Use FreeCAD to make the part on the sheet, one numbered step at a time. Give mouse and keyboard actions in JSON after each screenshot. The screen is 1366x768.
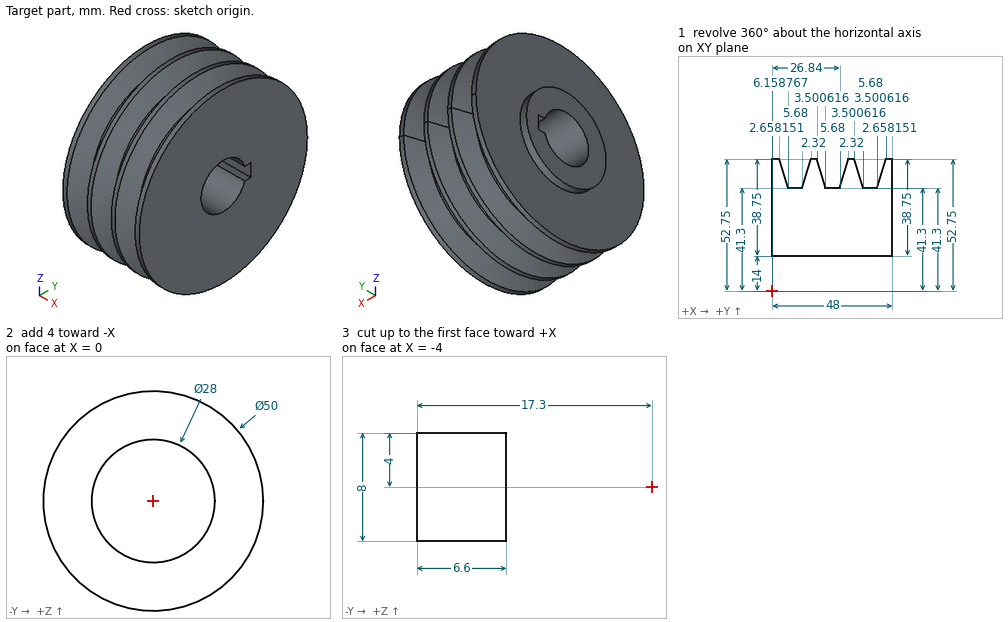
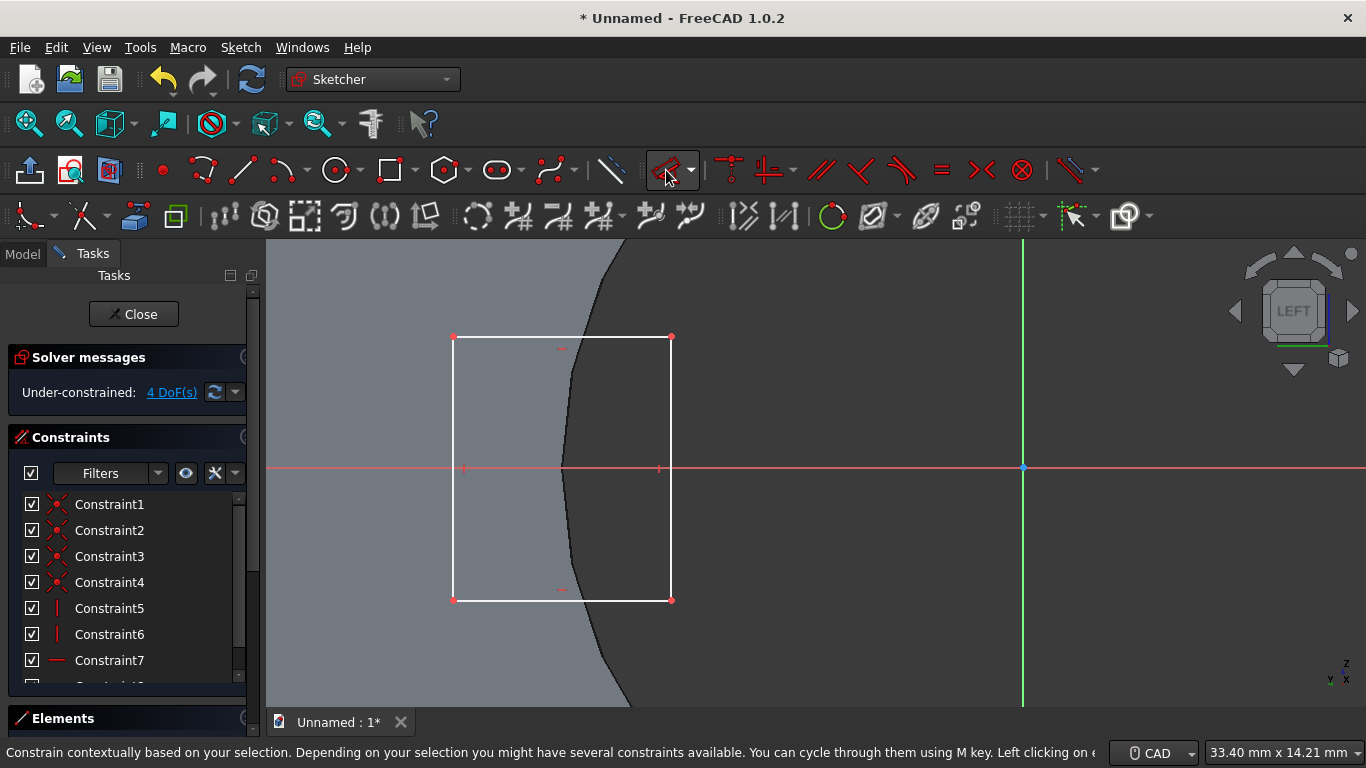
{"action": "left_click", "coordinate": [453, 416]}
{"action": "left_click", "coordinate": [419, 408]}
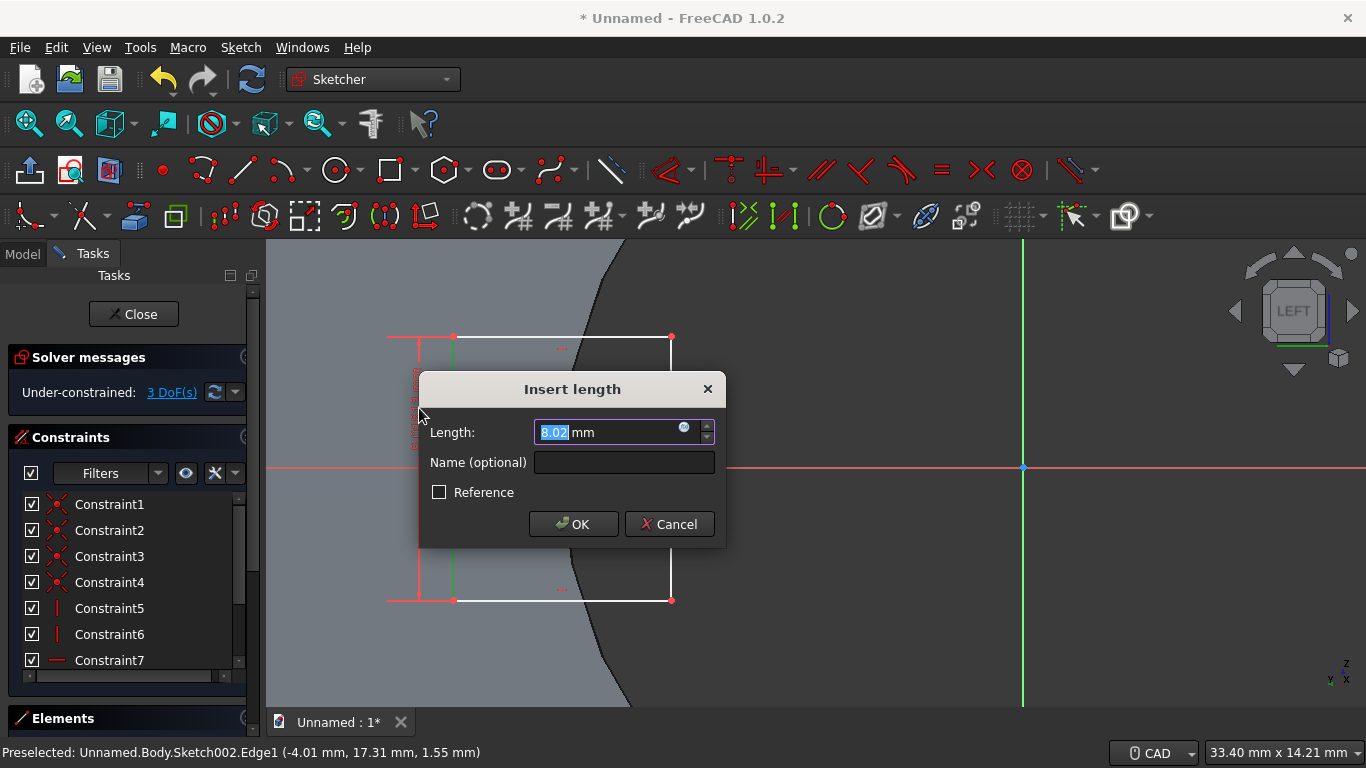
{"action": "type", "text": "8"}
{"action": "key", "text": "Return"}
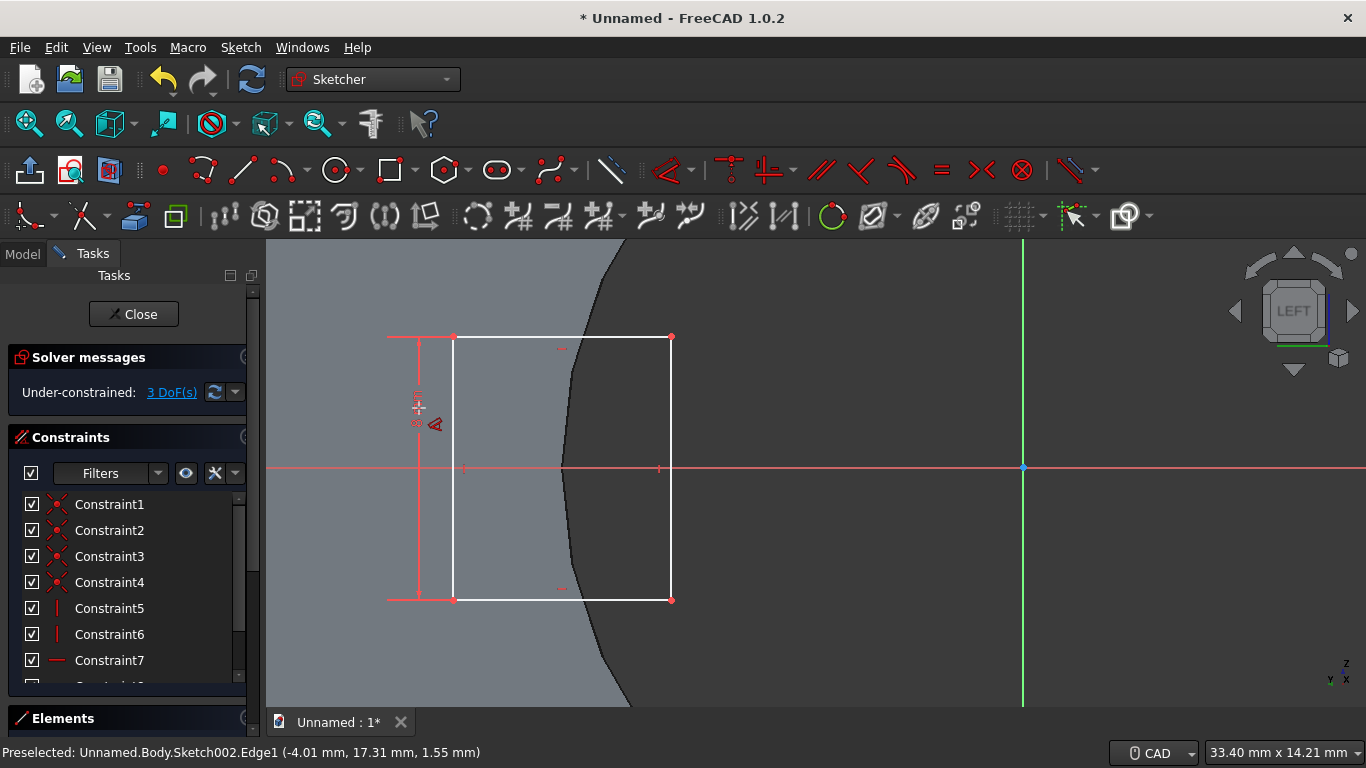
{"action": "left_click", "coordinate": [453, 337]}
{"action": "left_click", "coordinate": [419, 372]}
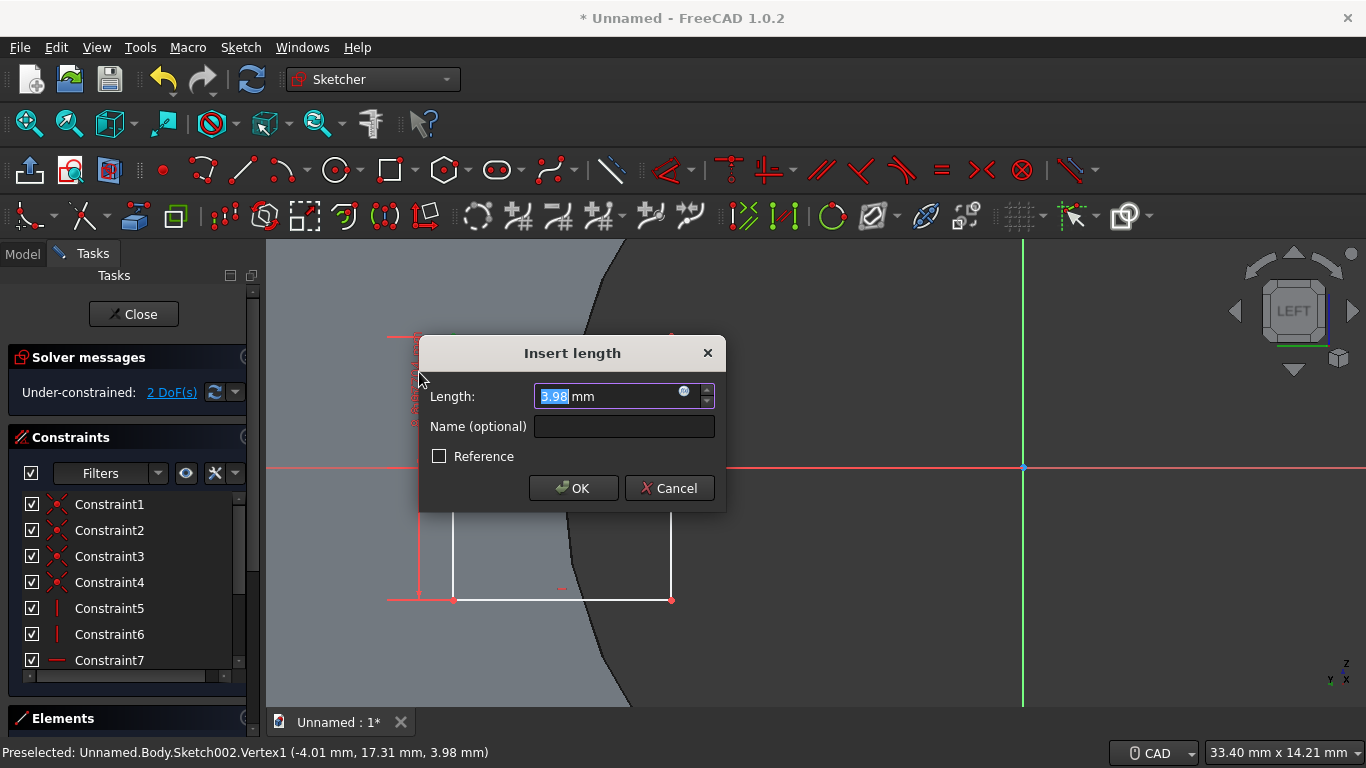
{"action": "type", "text": "4"}
{"action": "key", "text": "Return"}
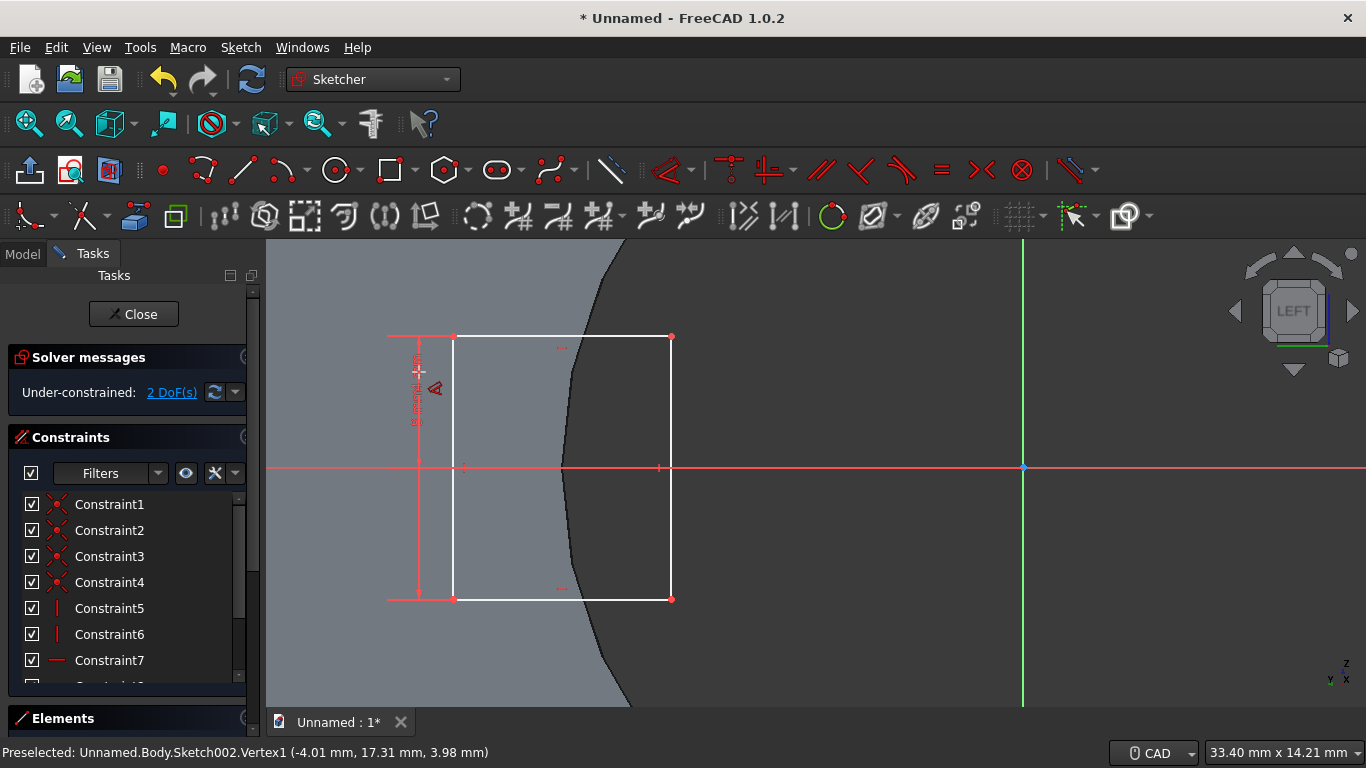
{"action": "left_click", "coordinate": [518, 600]}
{"action": "left_click", "coordinate": [562, 634]}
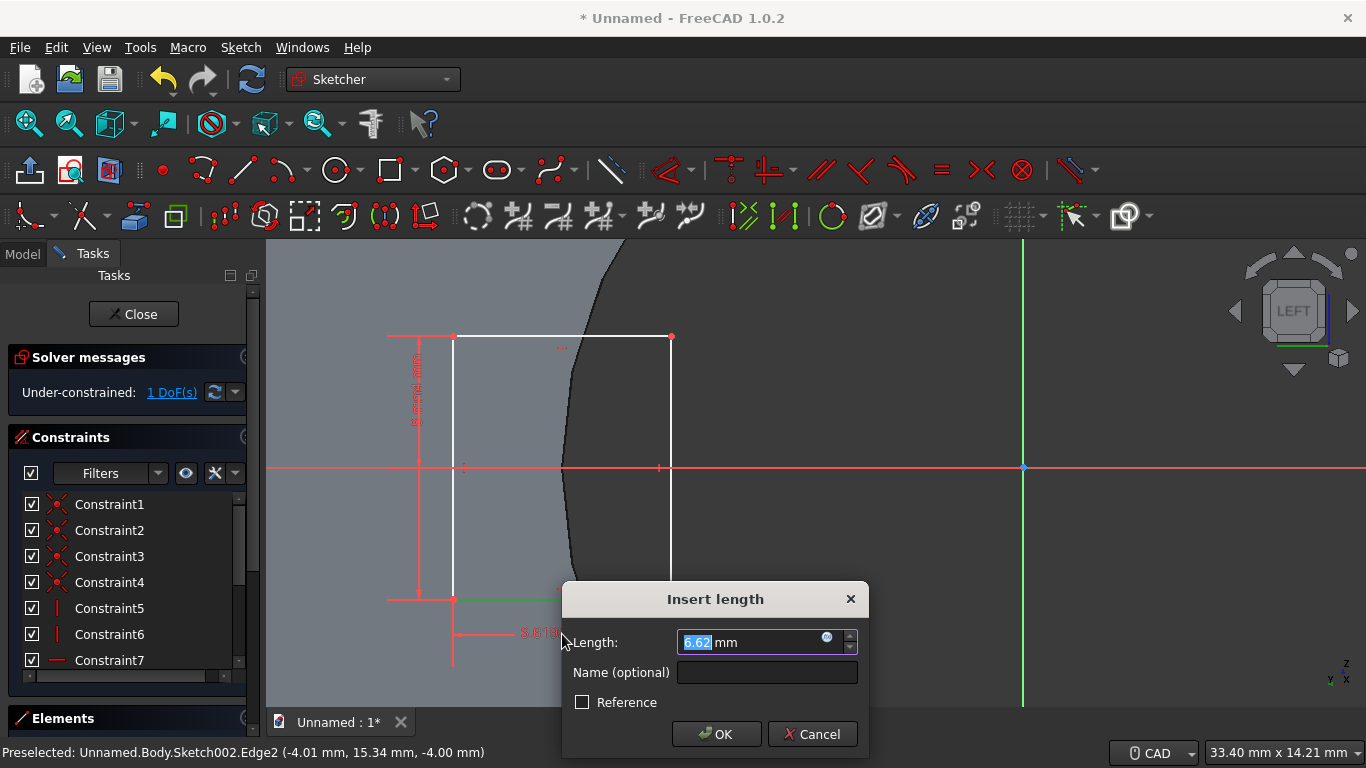
{"action": "type", "text": "6.6"}
{"action": "key", "text": "Return"}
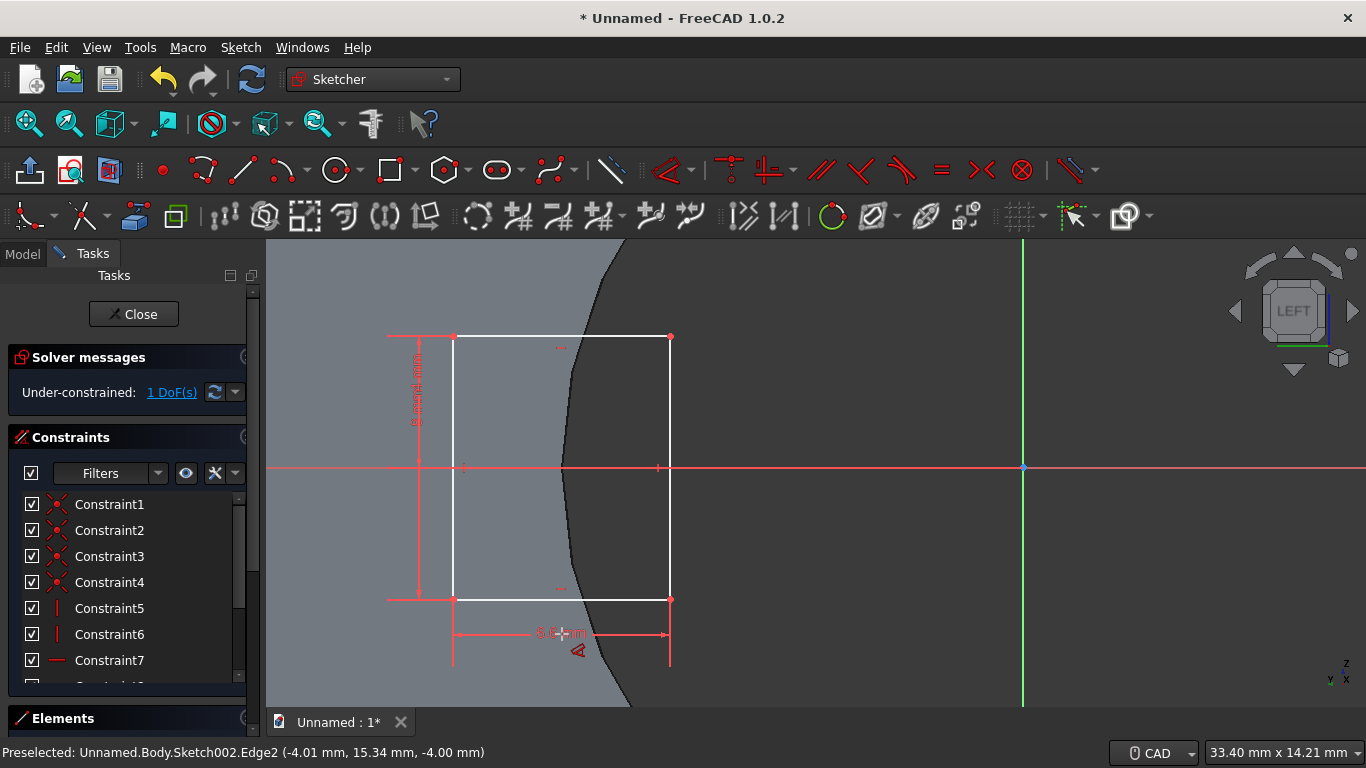
{"action": "left_click", "coordinate": [453, 336]}
{"action": "left_click", "coordinate": [738, 302]}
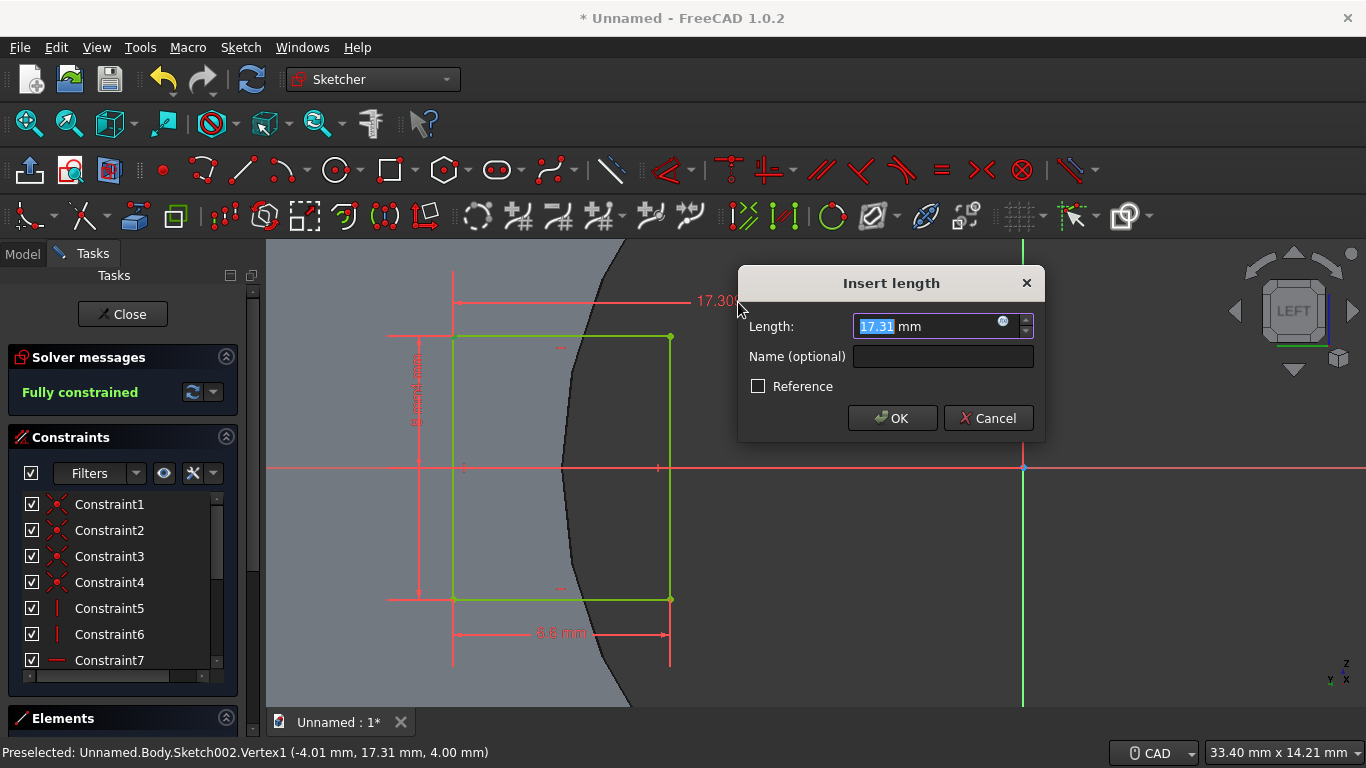
{"action": "type", "text": "17.3"}
{"action": "key", "text": "Return"}
{"action": "key", "text": "Escape"}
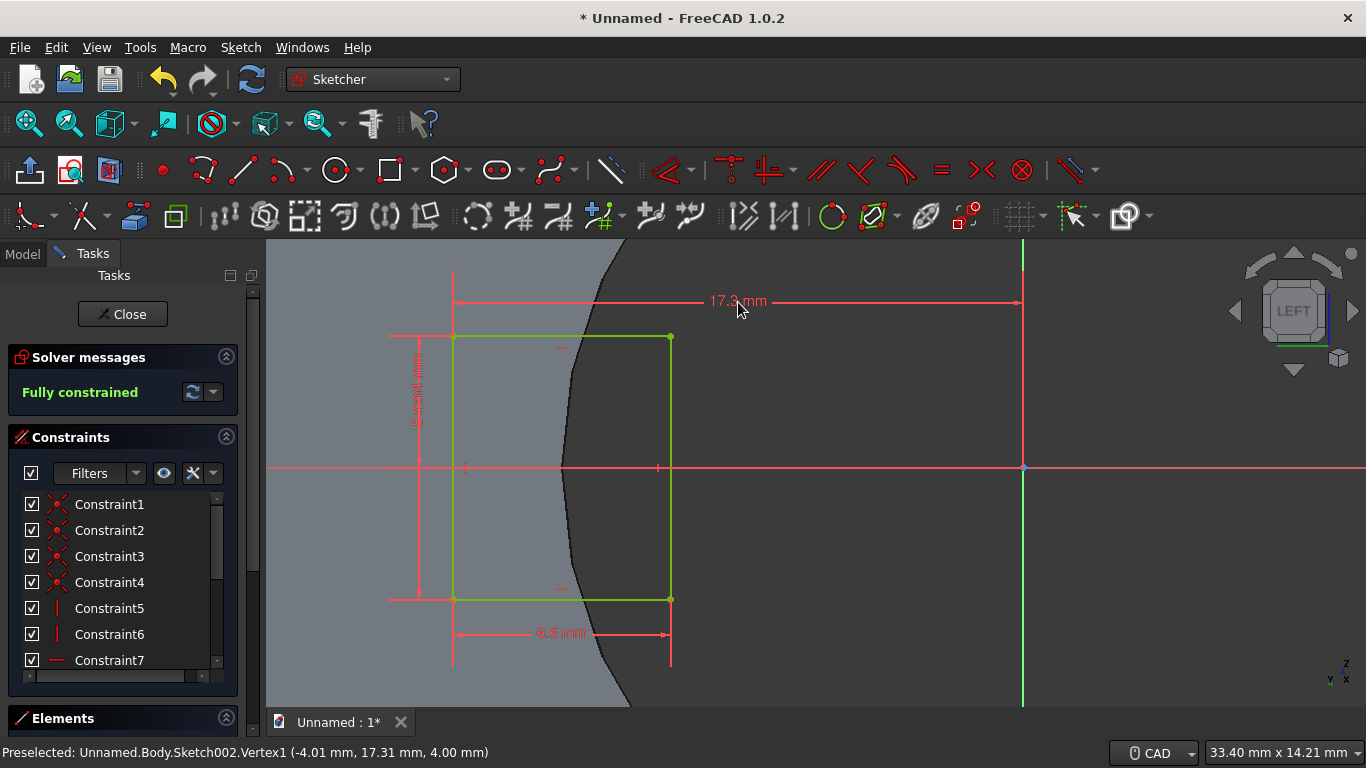
{"action": "left_click", "coordinate": [123, 314]}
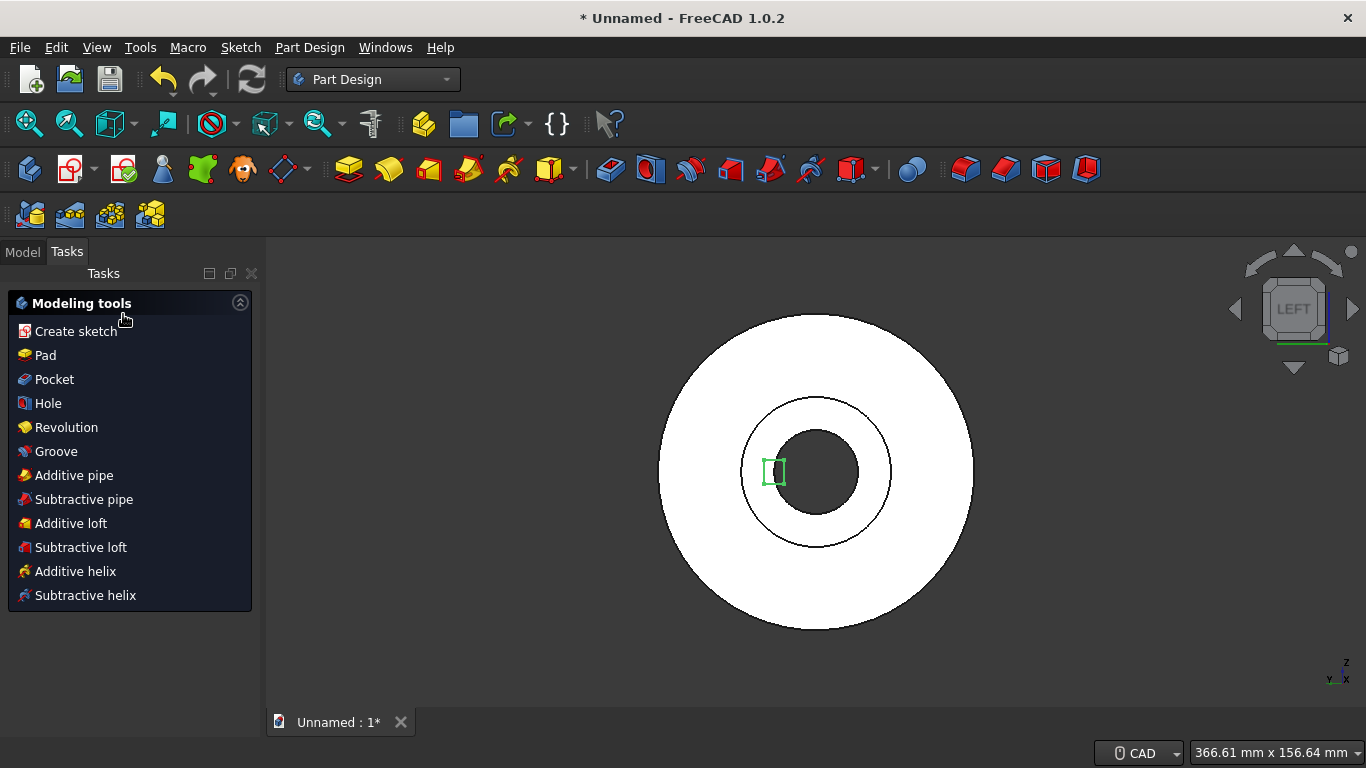
{"action": "left_click", "coordinate": [612, 170]}